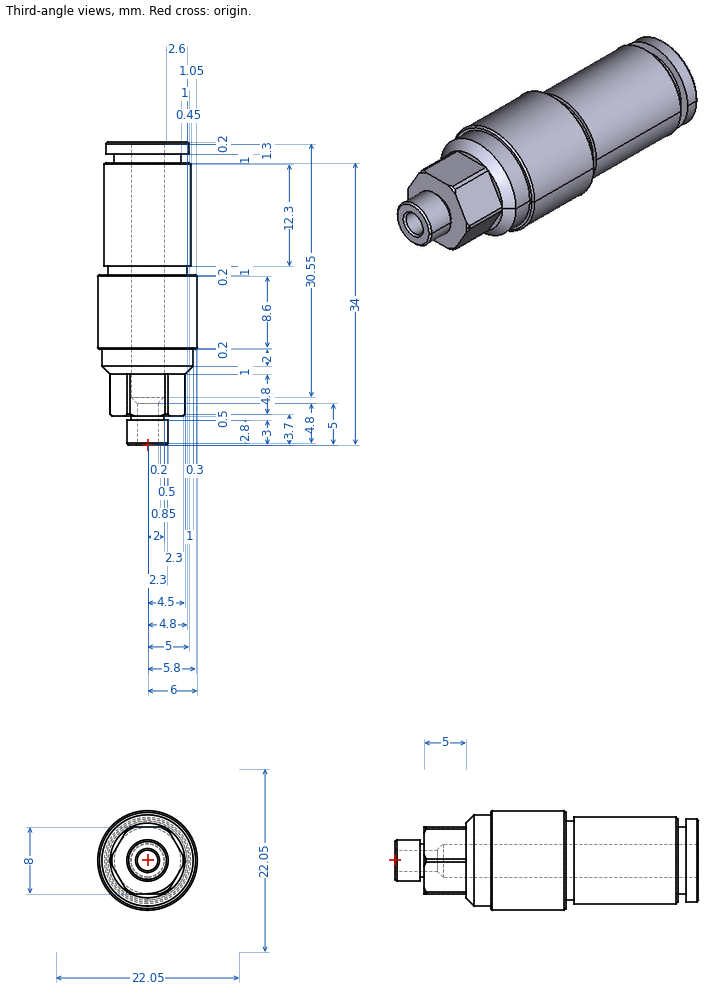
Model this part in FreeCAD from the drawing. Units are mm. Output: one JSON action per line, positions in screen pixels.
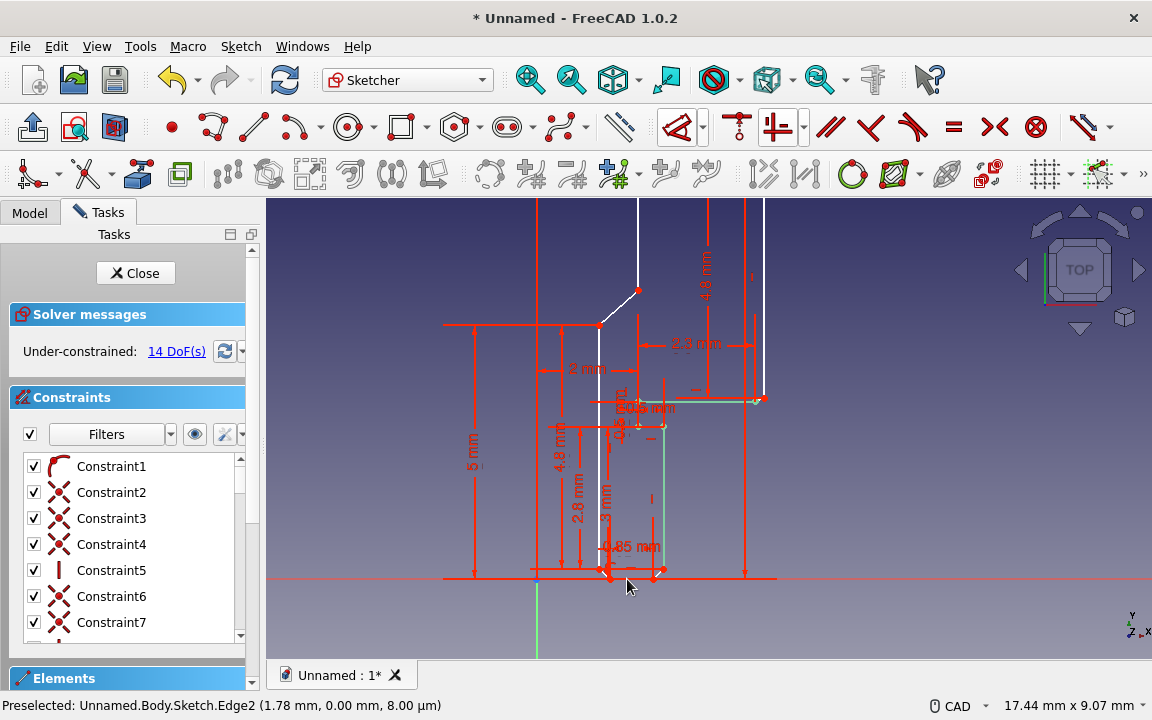
{"action": "scroll", "coordinate": [631, 582], "scroll_direction": "down", "scroll_amount": 9}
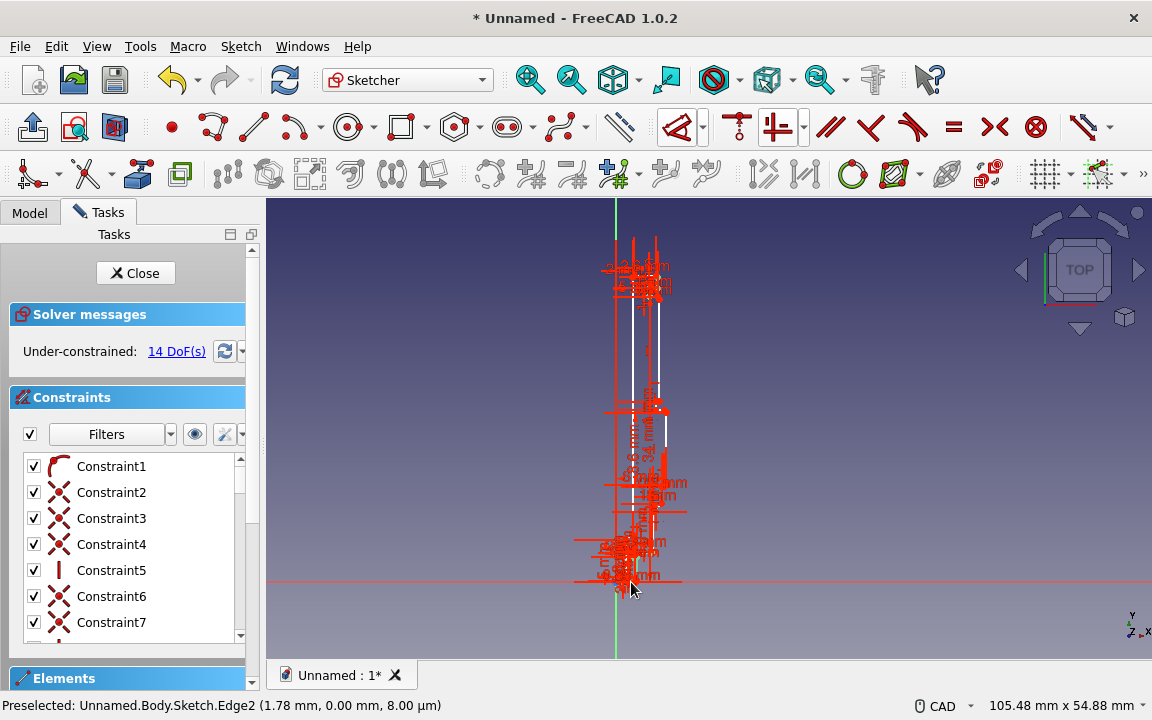
{"action": "scroll", "coordinate": [662, 410], "scroll_direction": "up", "scroll_amount": 9}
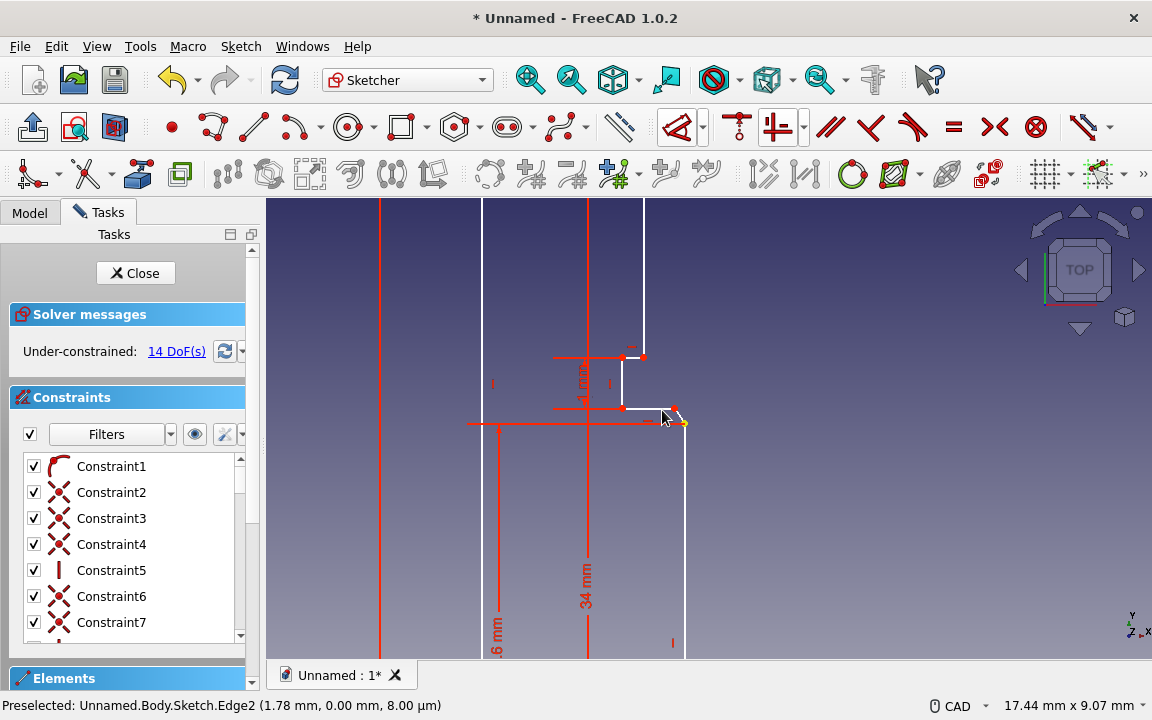
{"action": "left_click", "coordinate": [659, 409]}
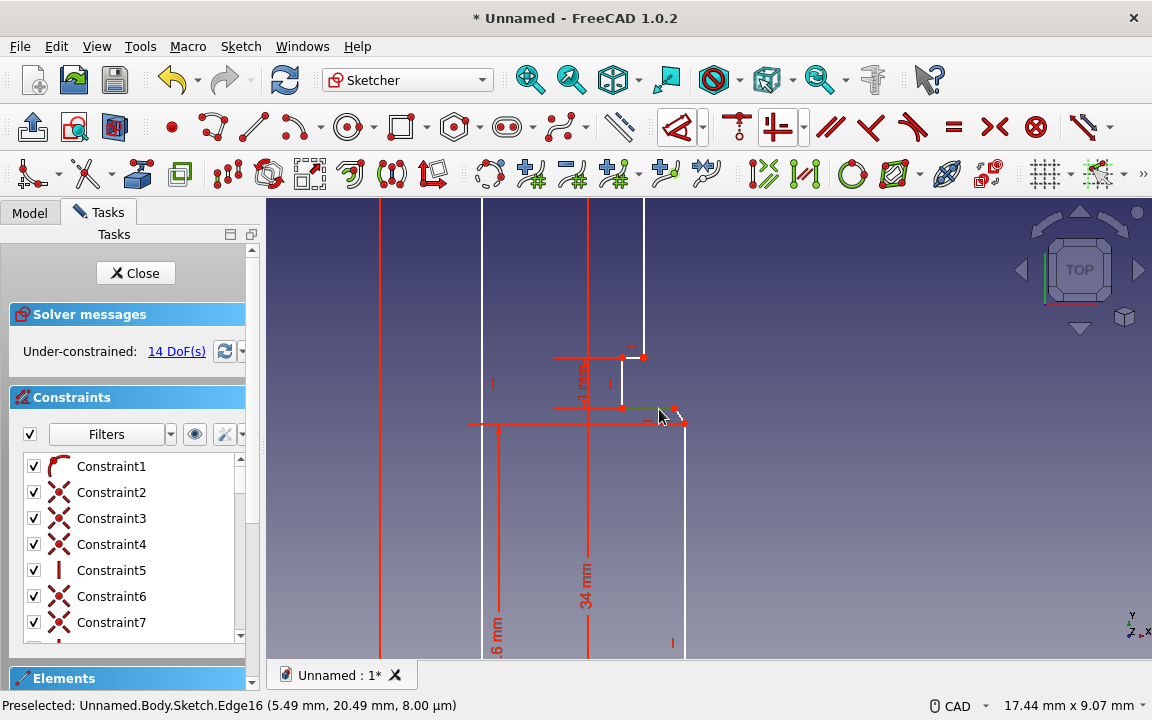
{"action": "key", "text": "l"}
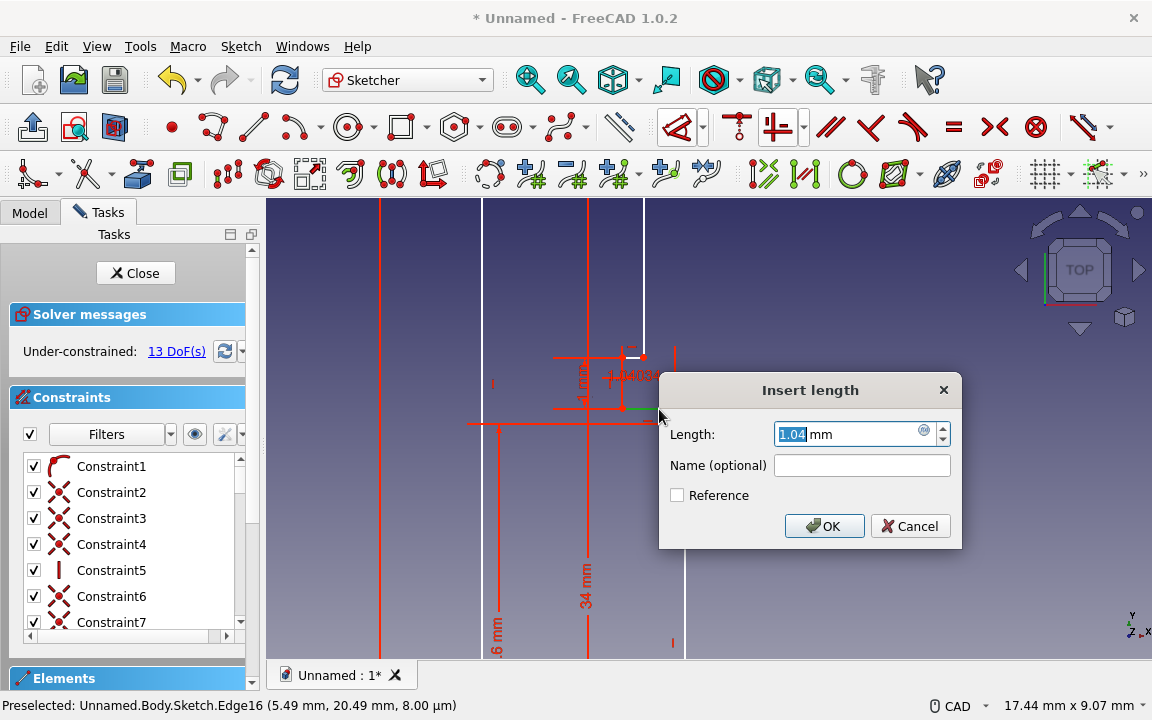
{"action": "type", "text": "1.05"}
{"action": "key", "text": "Return"}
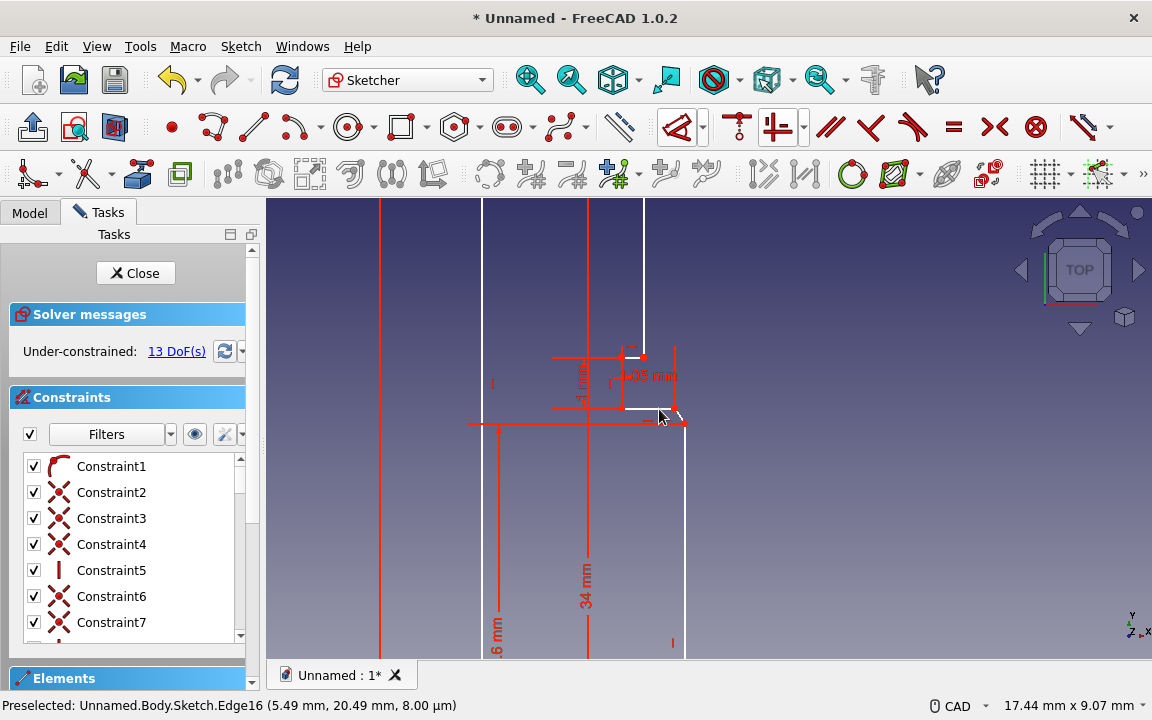
{"action": "scroll", "coordinate": [633, 358], "scroll_direction": "up", "scroll_amount": 3}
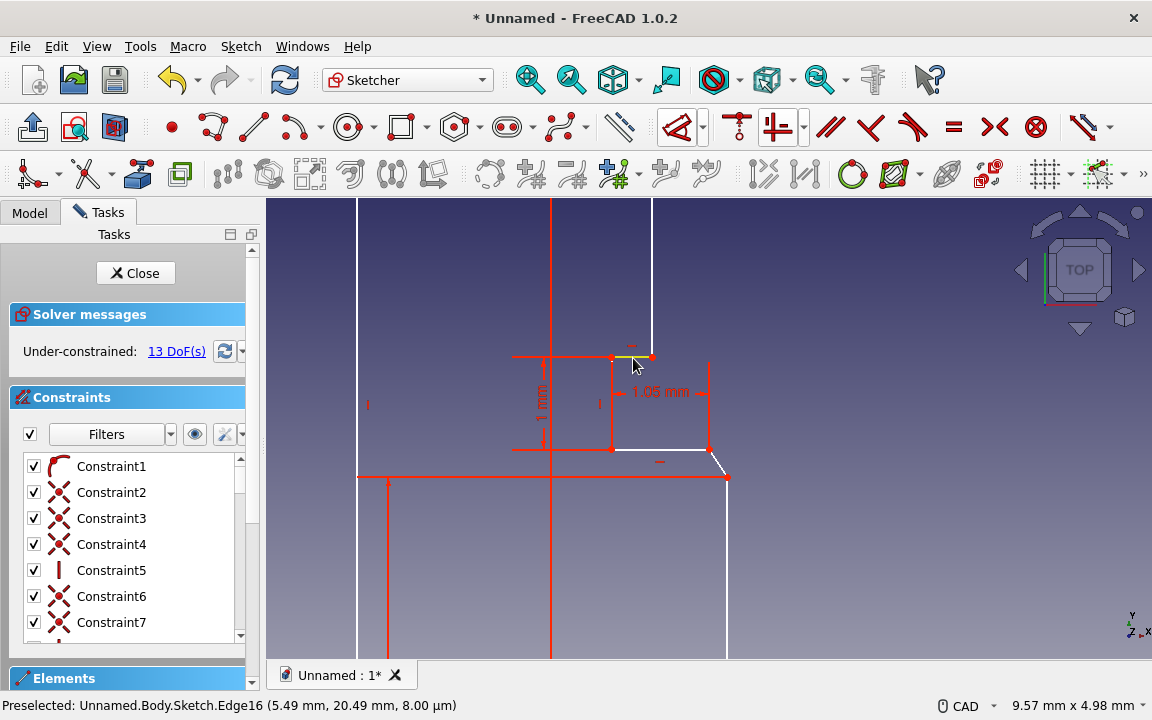
{"action": "left_click", "coordinate": [632, 357]}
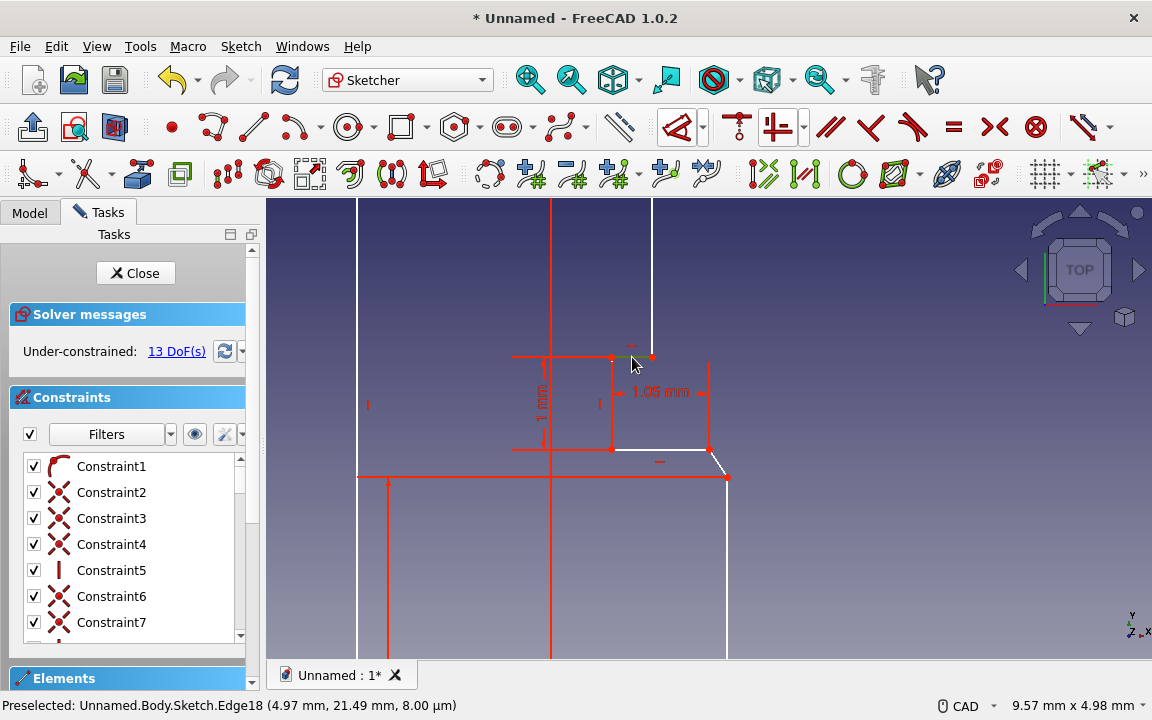
{"action": "key", "text": "l"}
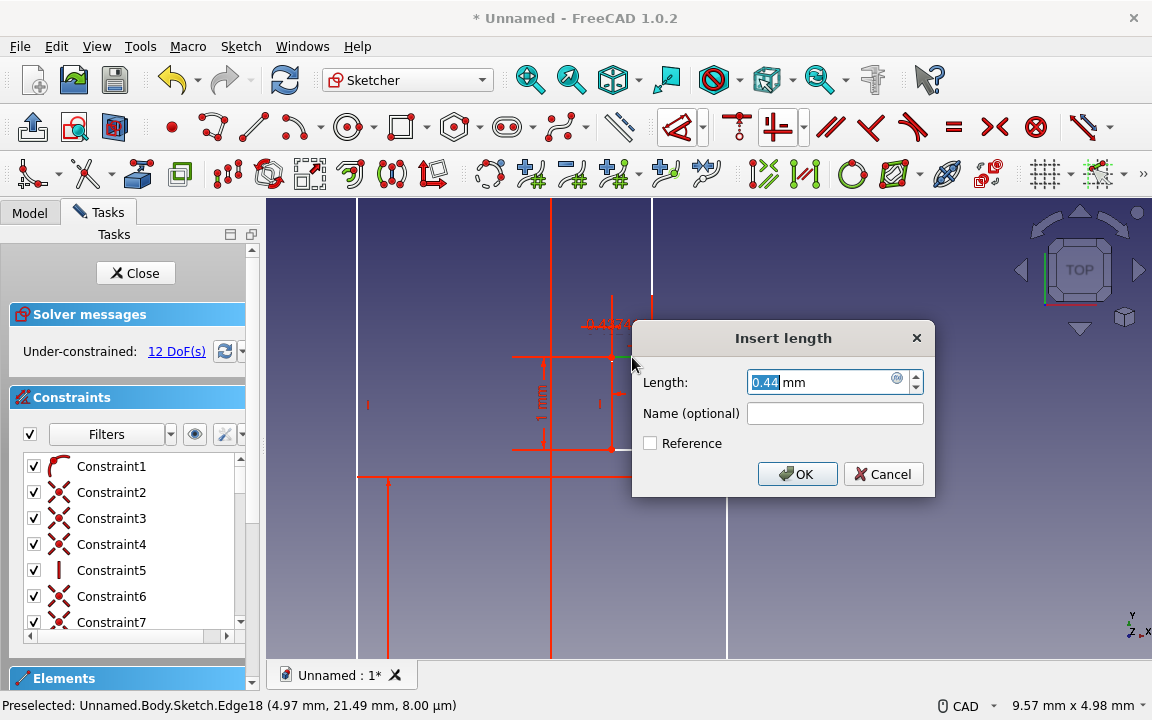
{"action": "type", "text": "0.45"}
{"action": "key", "text": "Return"}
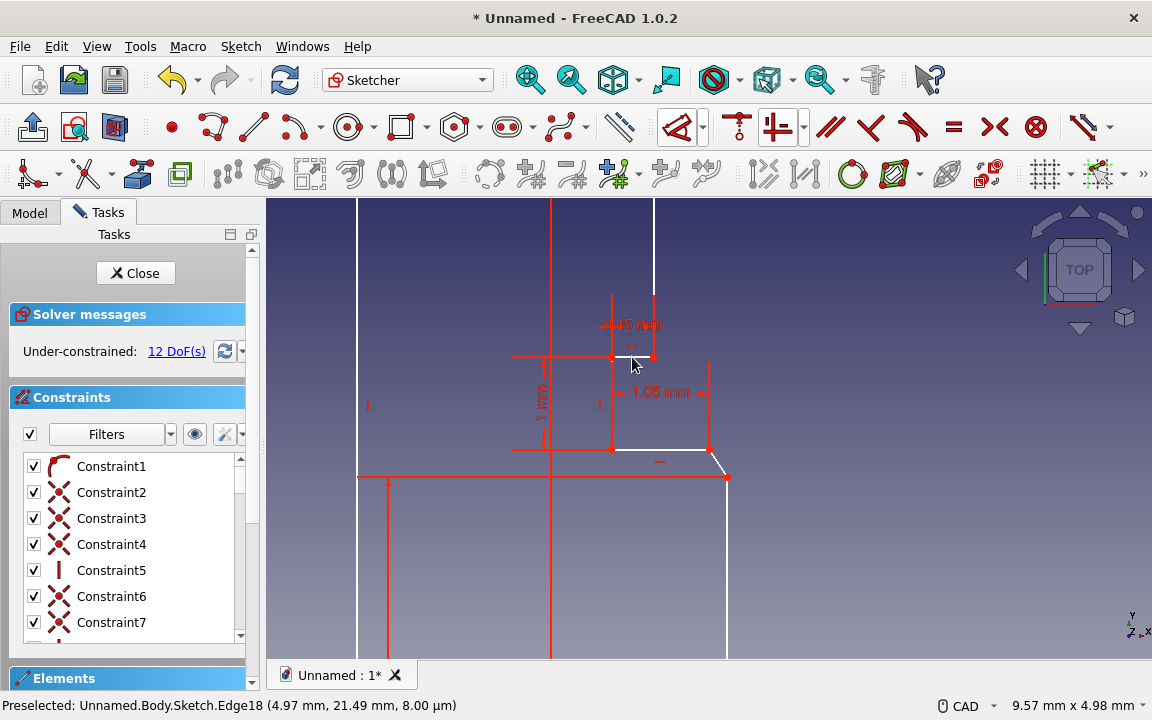
{"action": "scroll", "coordinate": [660, 406], "scroll_direction": "down", "scroll_amount": 12}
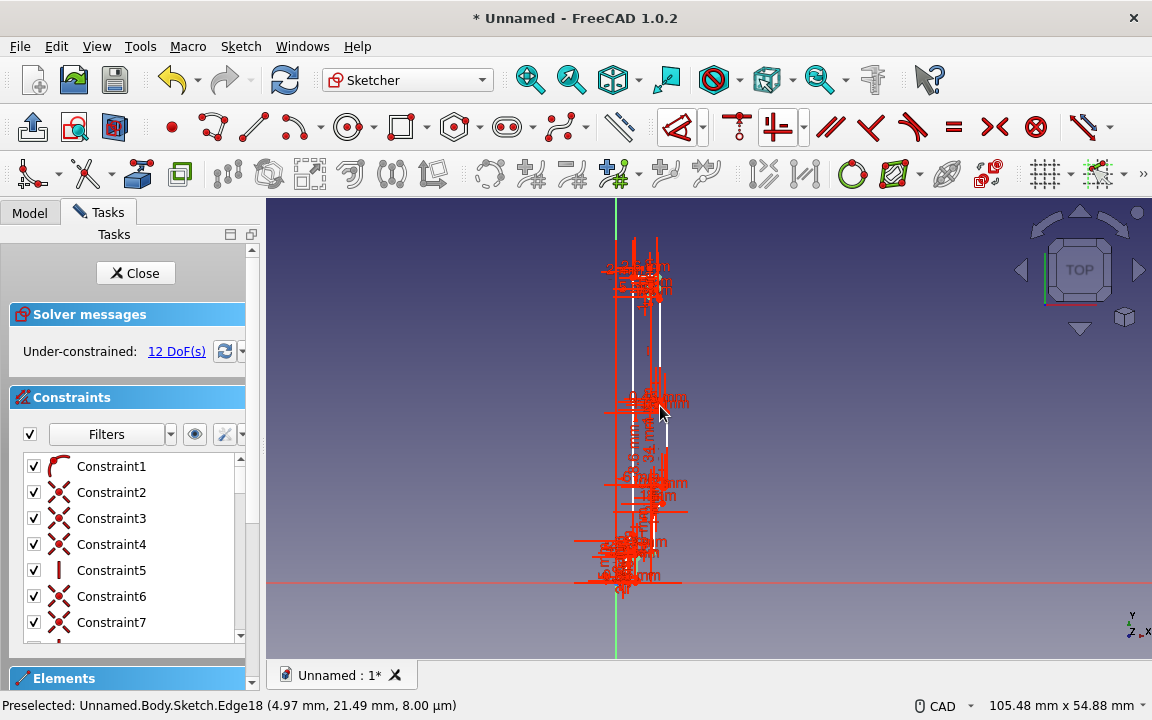
{"action": "left_click", "coordinate": [660, 371]}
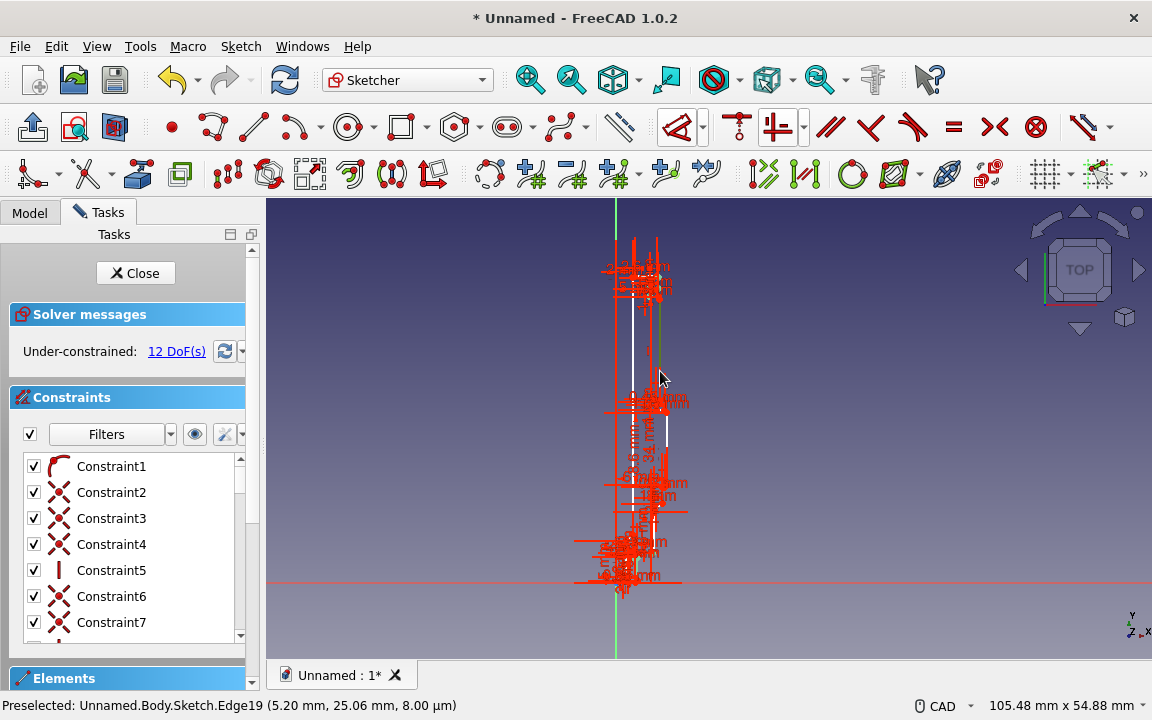
{"action": "key", "text": "i"}